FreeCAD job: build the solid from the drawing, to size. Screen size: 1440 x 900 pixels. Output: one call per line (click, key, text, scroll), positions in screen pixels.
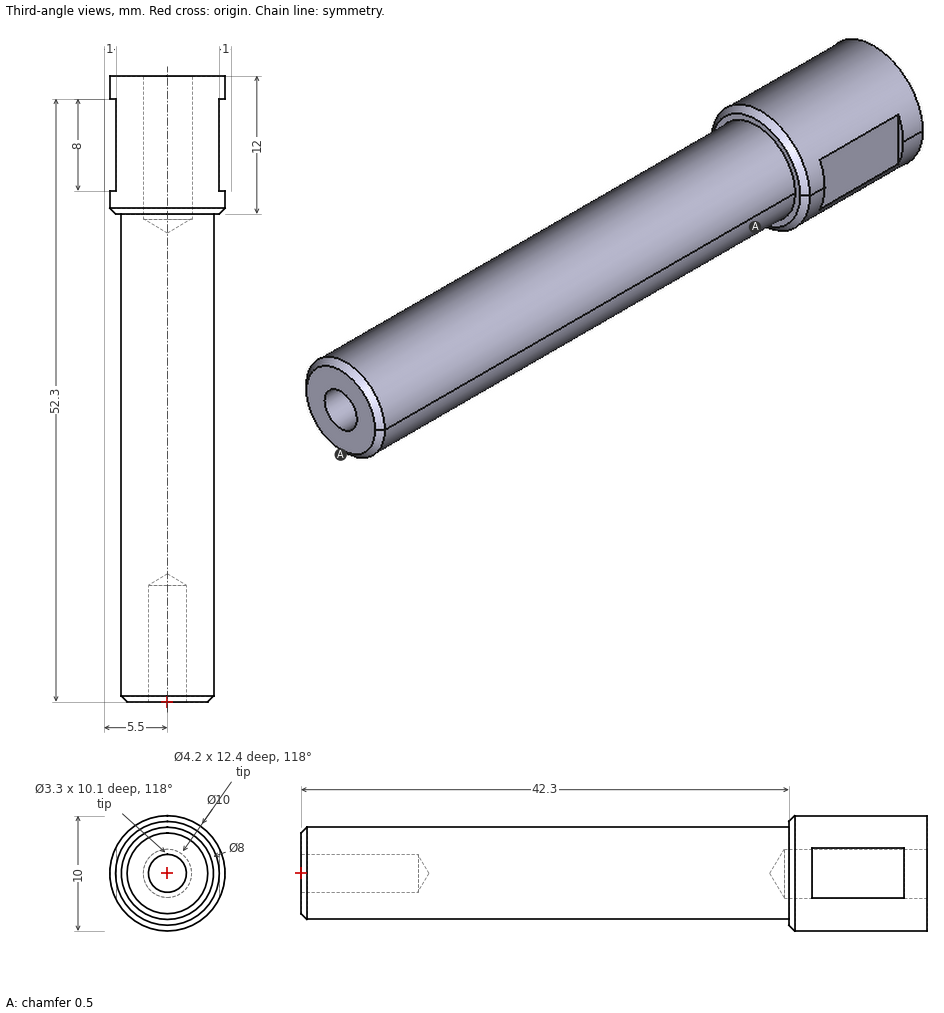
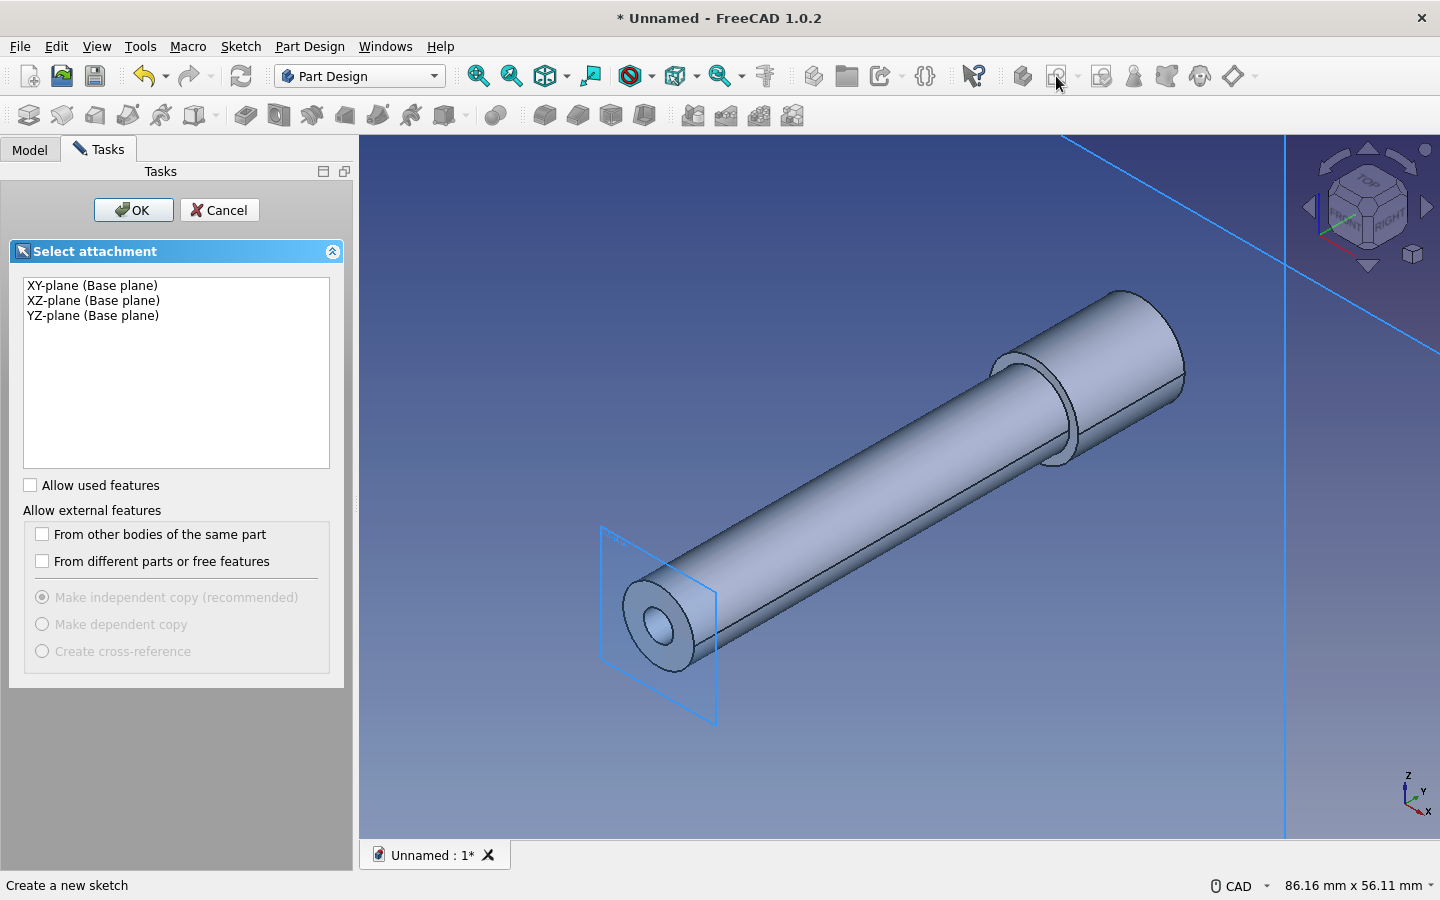
click(84, 286)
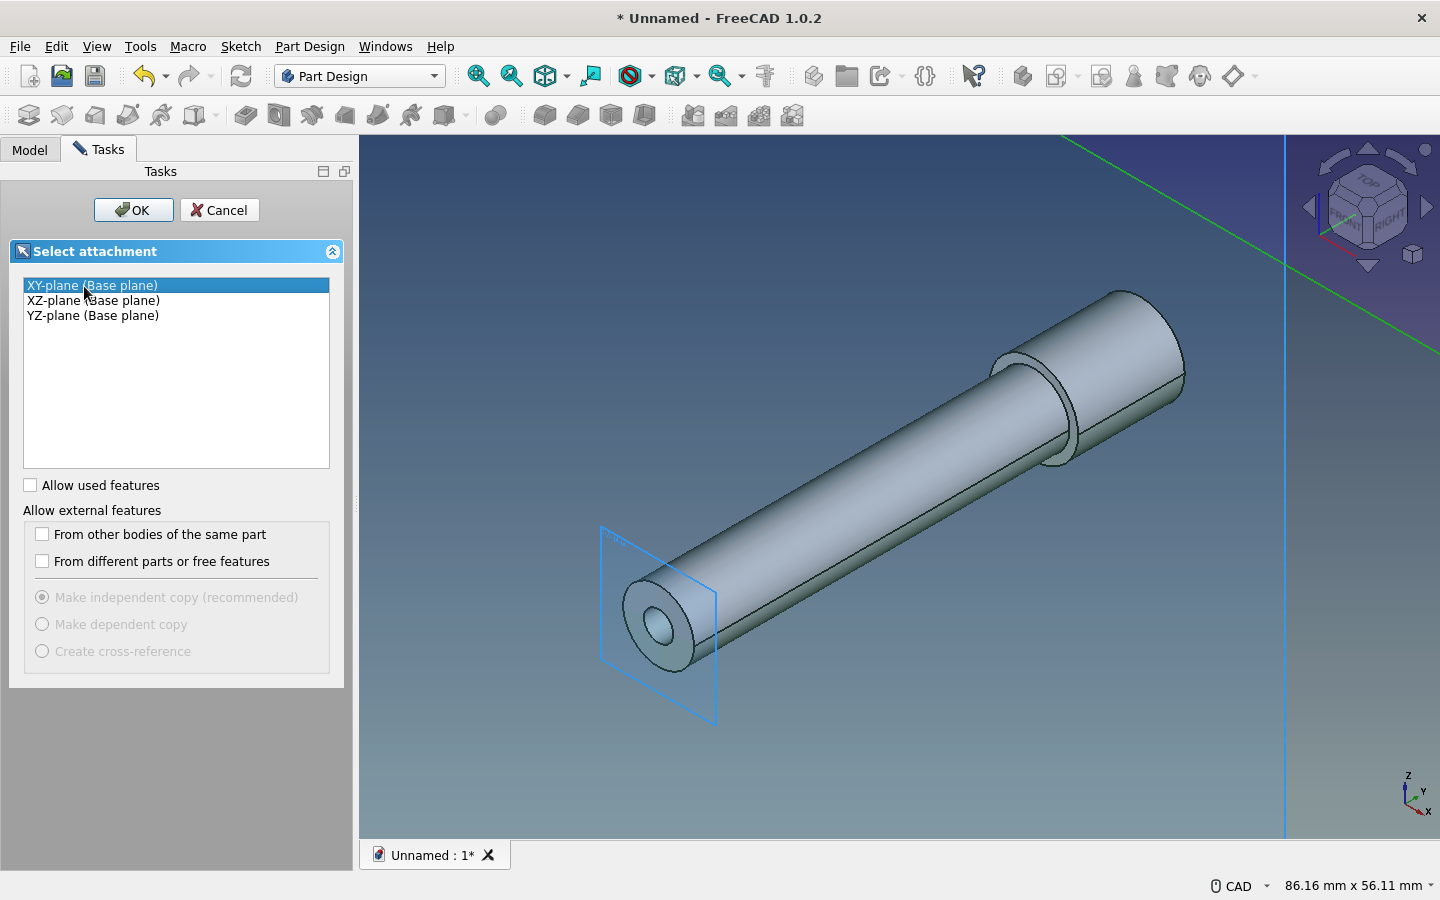
click(134, 210)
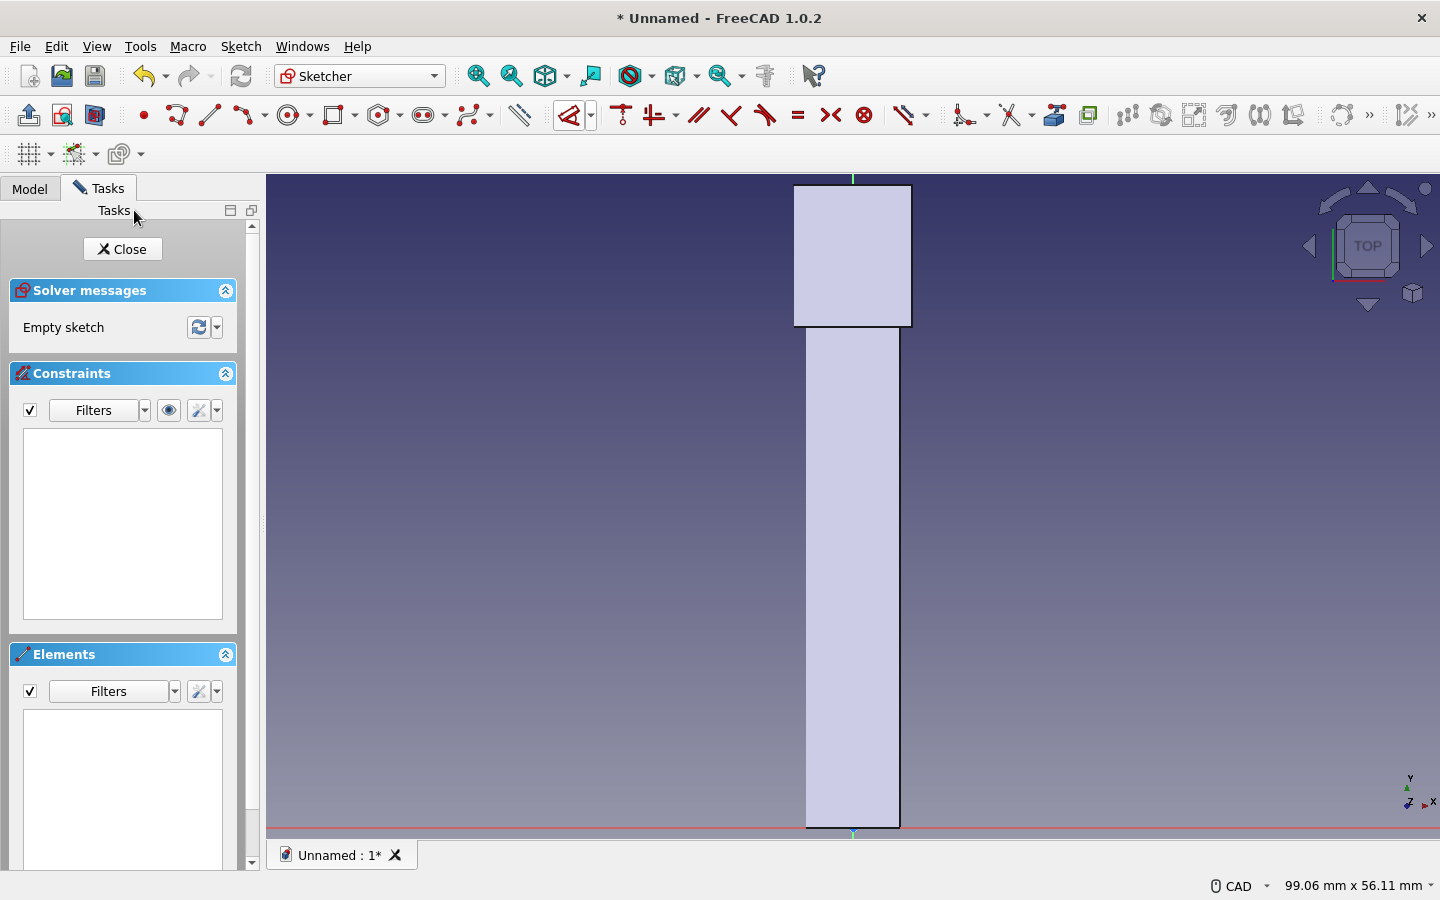
key(q)
key(s)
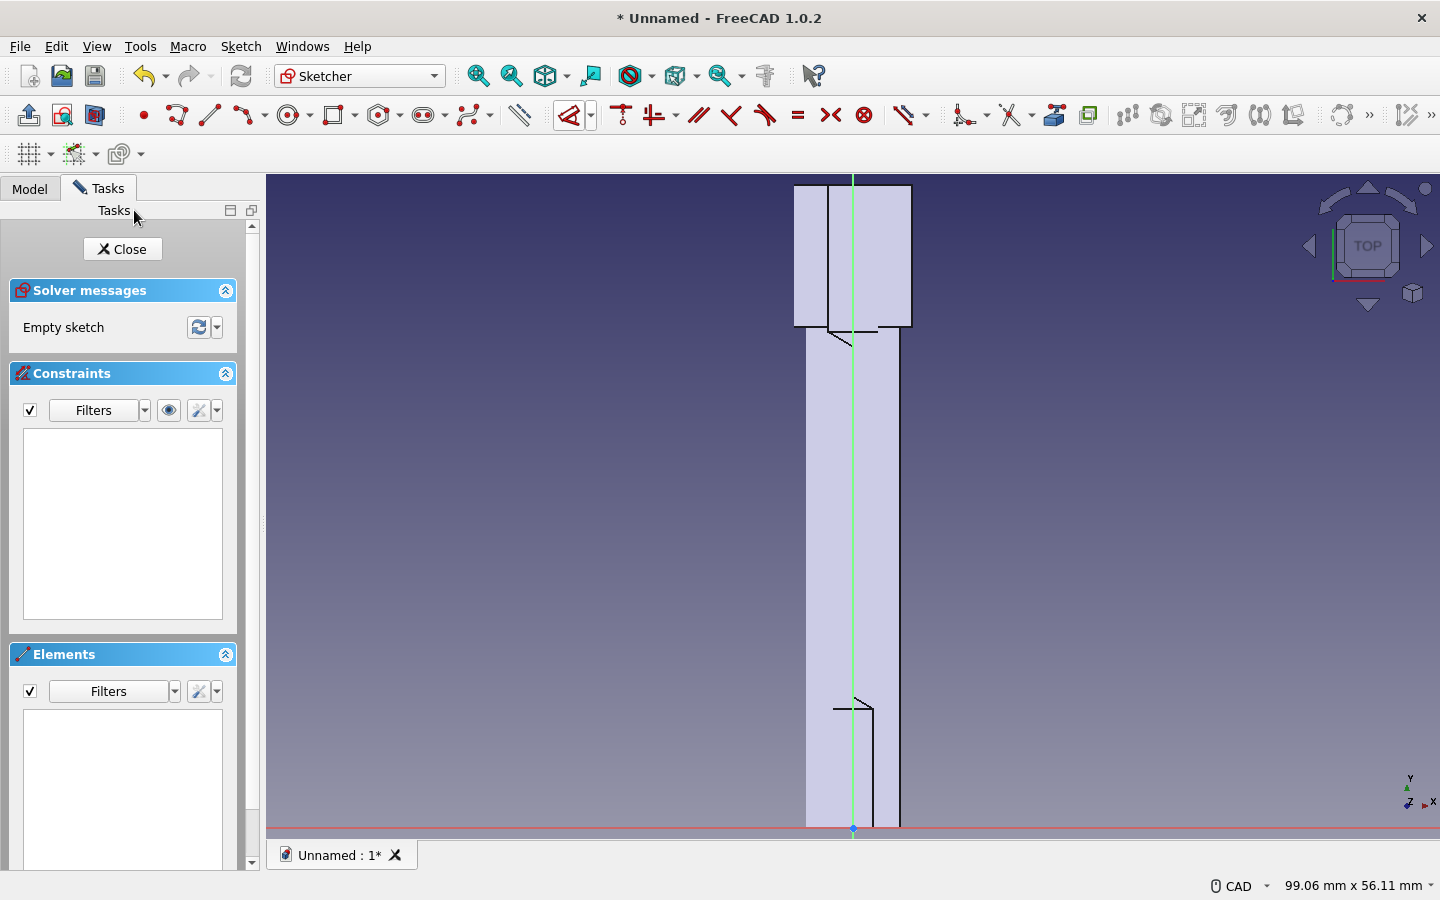
scroll(870, 202, up, 8)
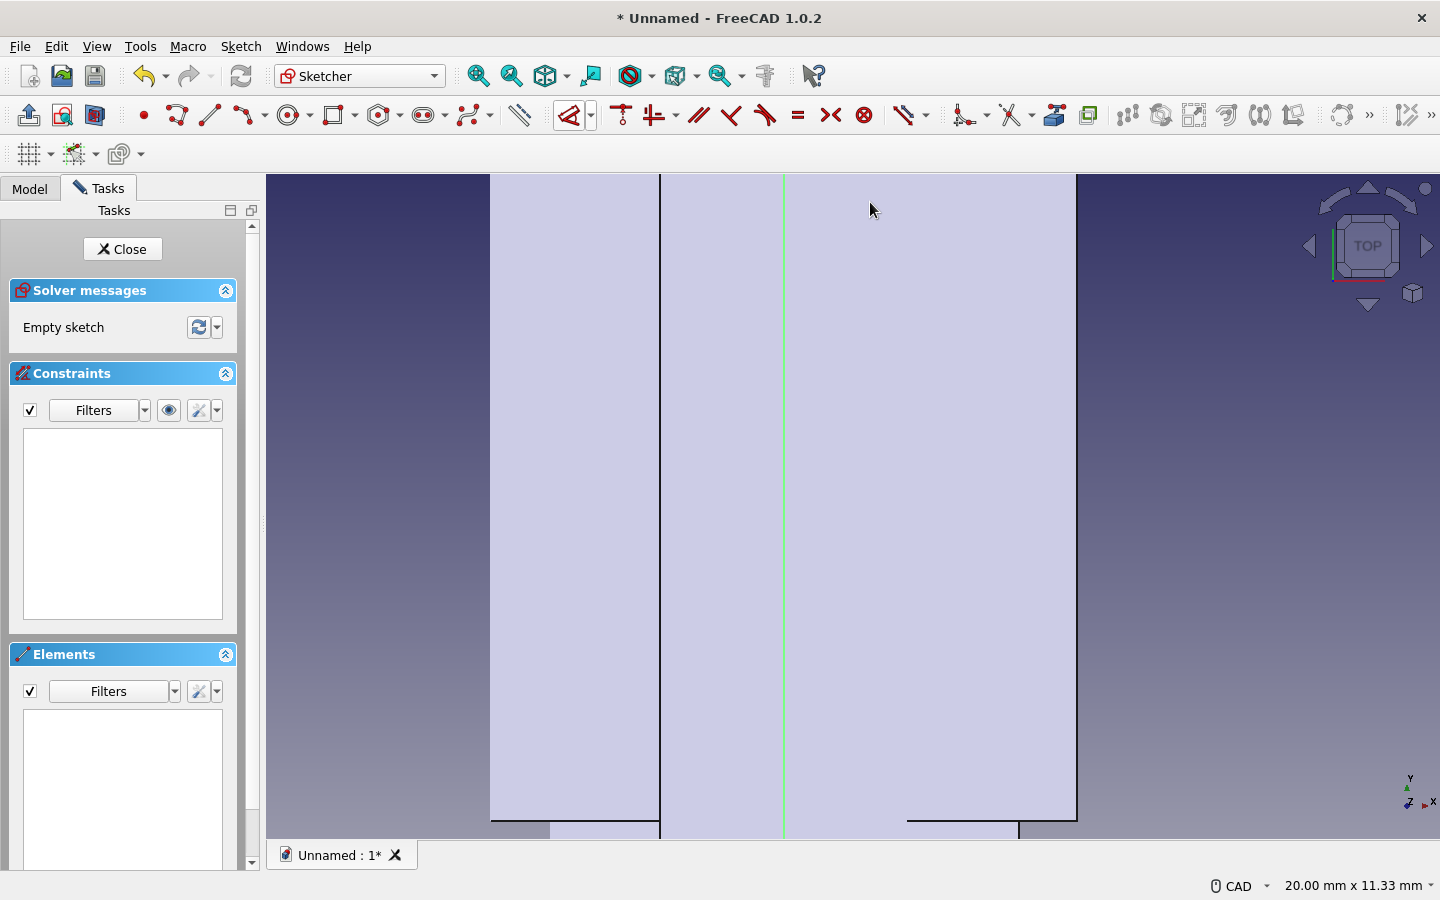
key(g)
key(r)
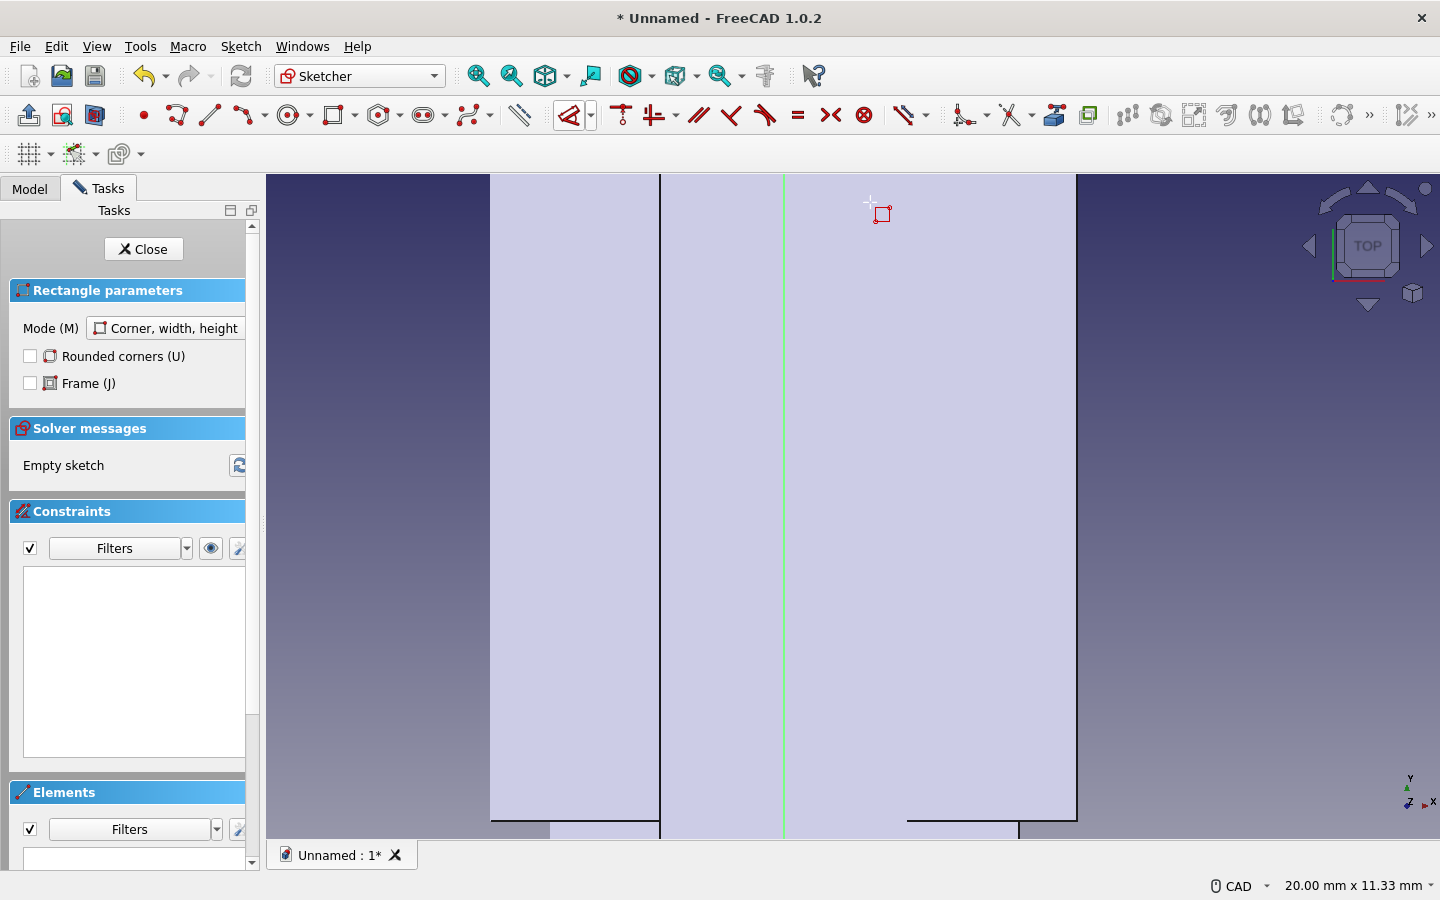
click(461, 234)
move(520, 703)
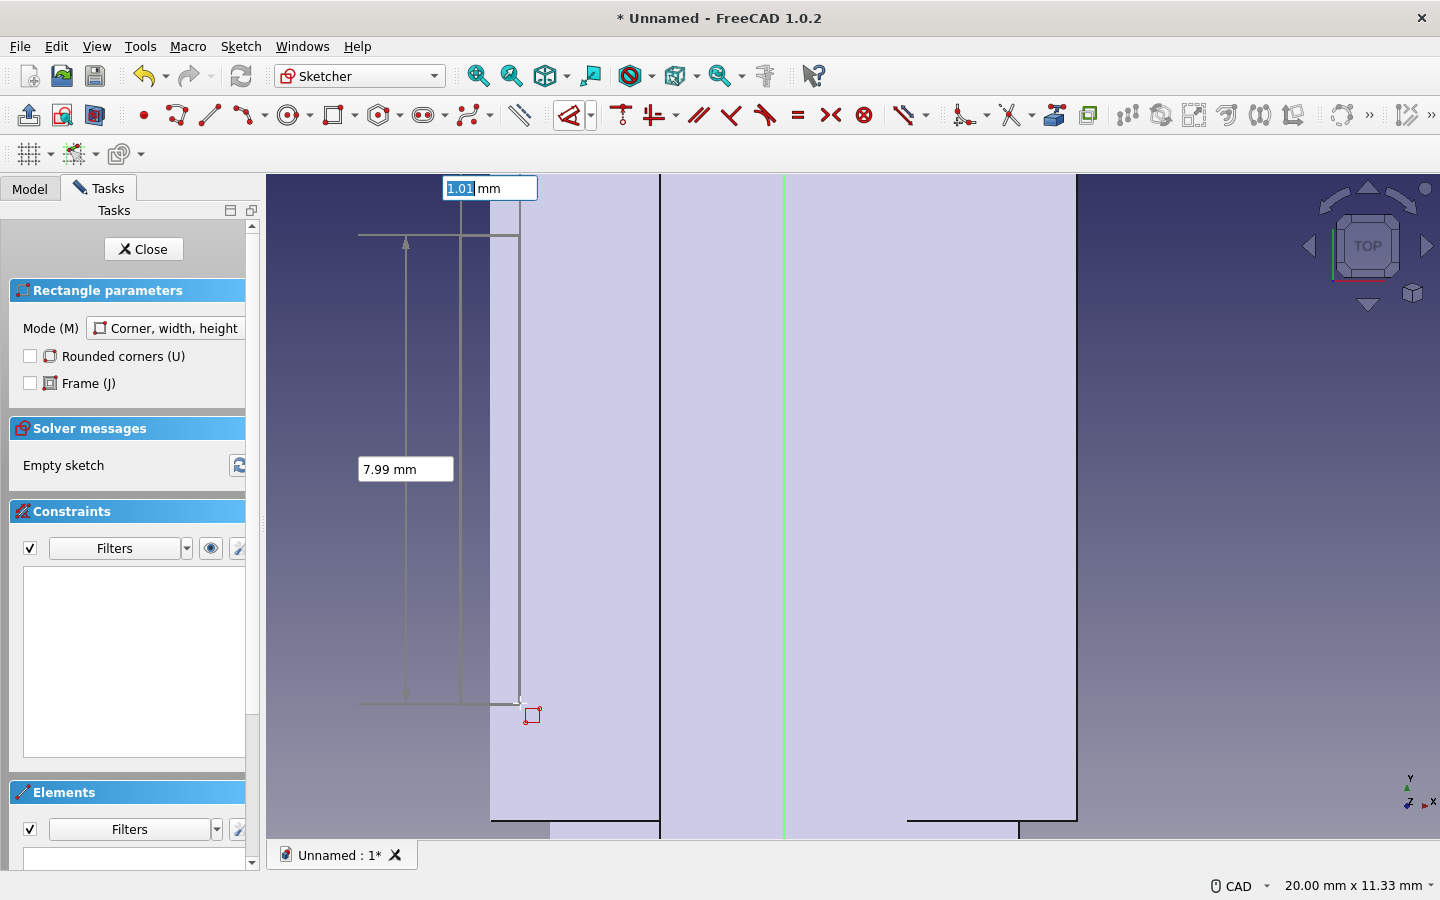
text(1)
key(Tab)
text(8)
key(Return)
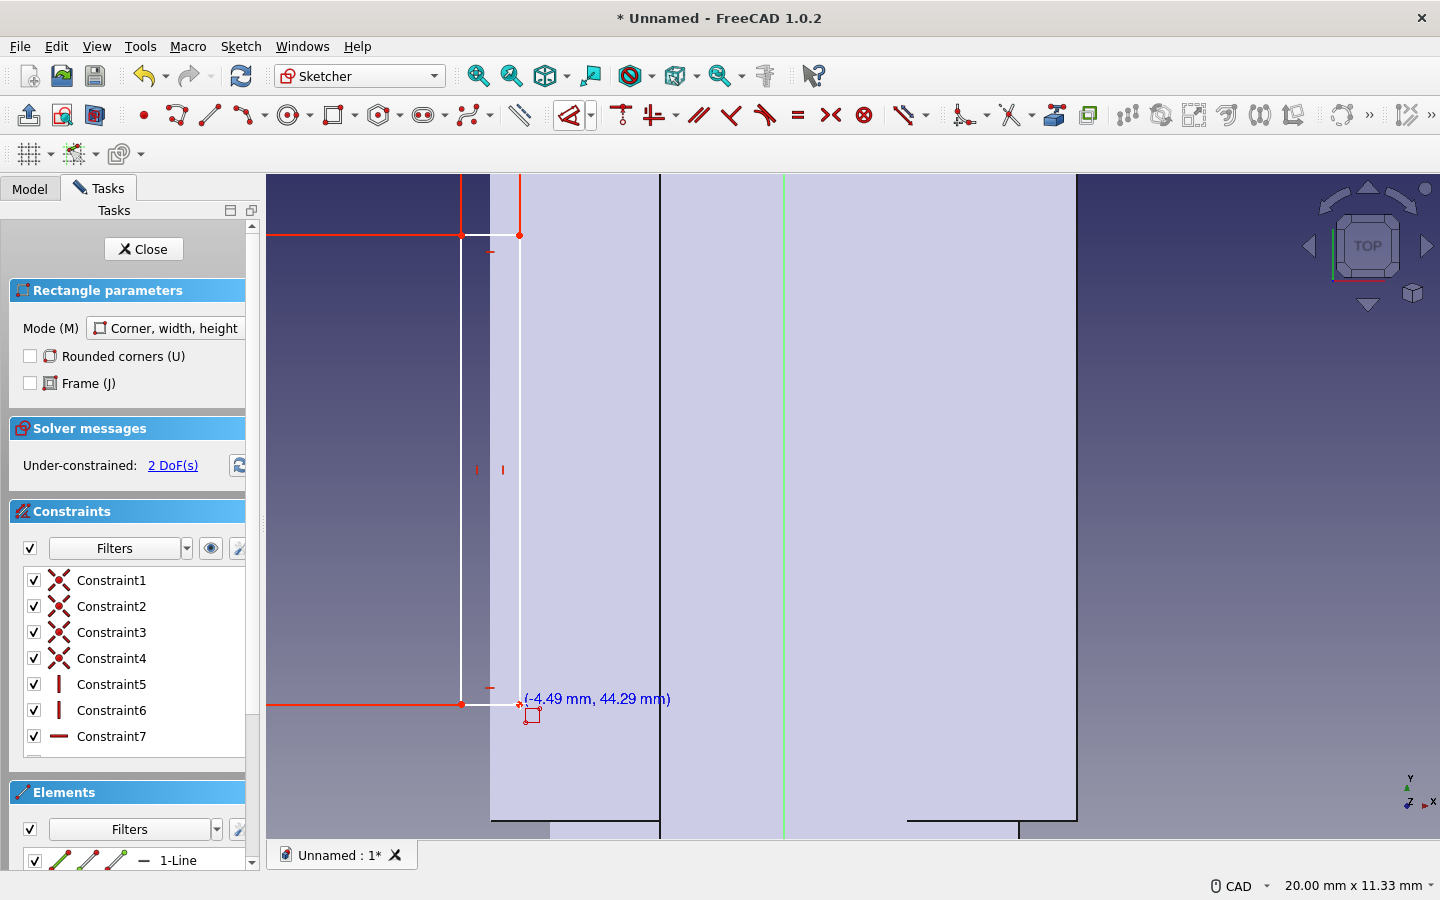
click(1048, 234)
move(1107, 703)